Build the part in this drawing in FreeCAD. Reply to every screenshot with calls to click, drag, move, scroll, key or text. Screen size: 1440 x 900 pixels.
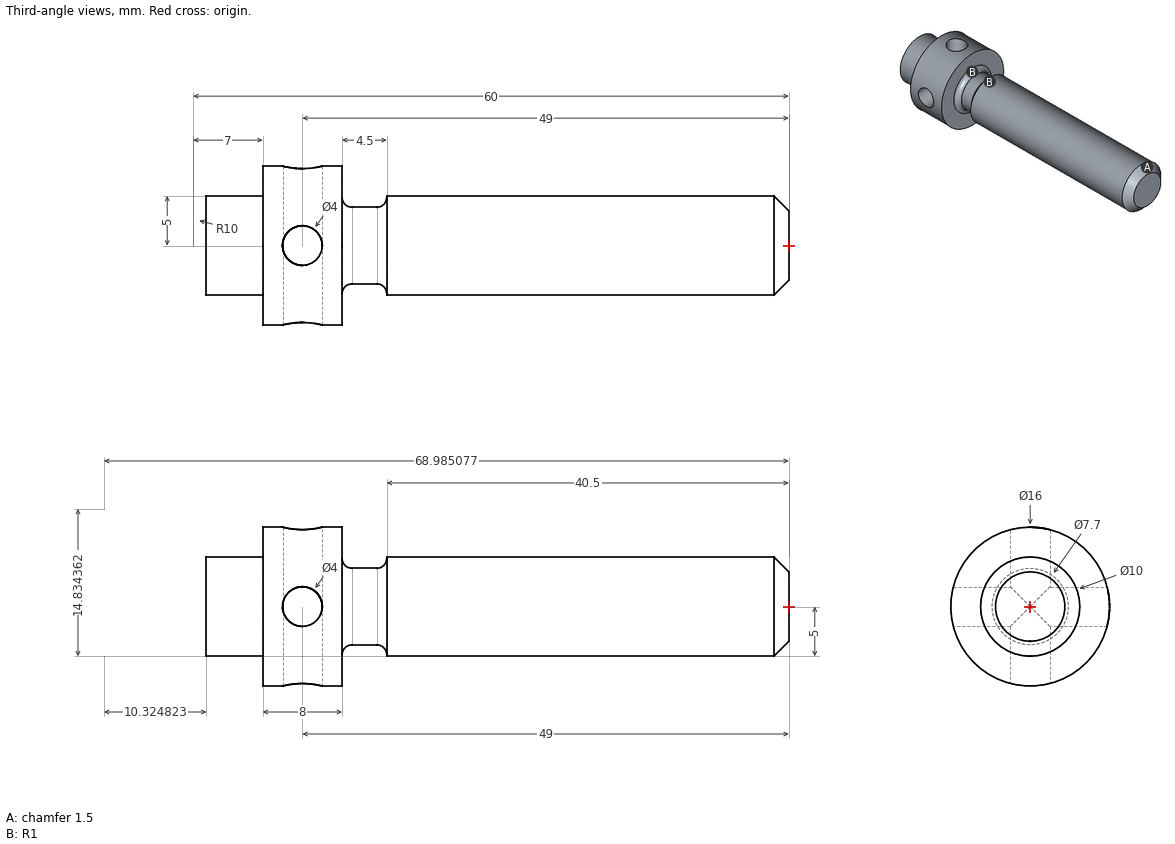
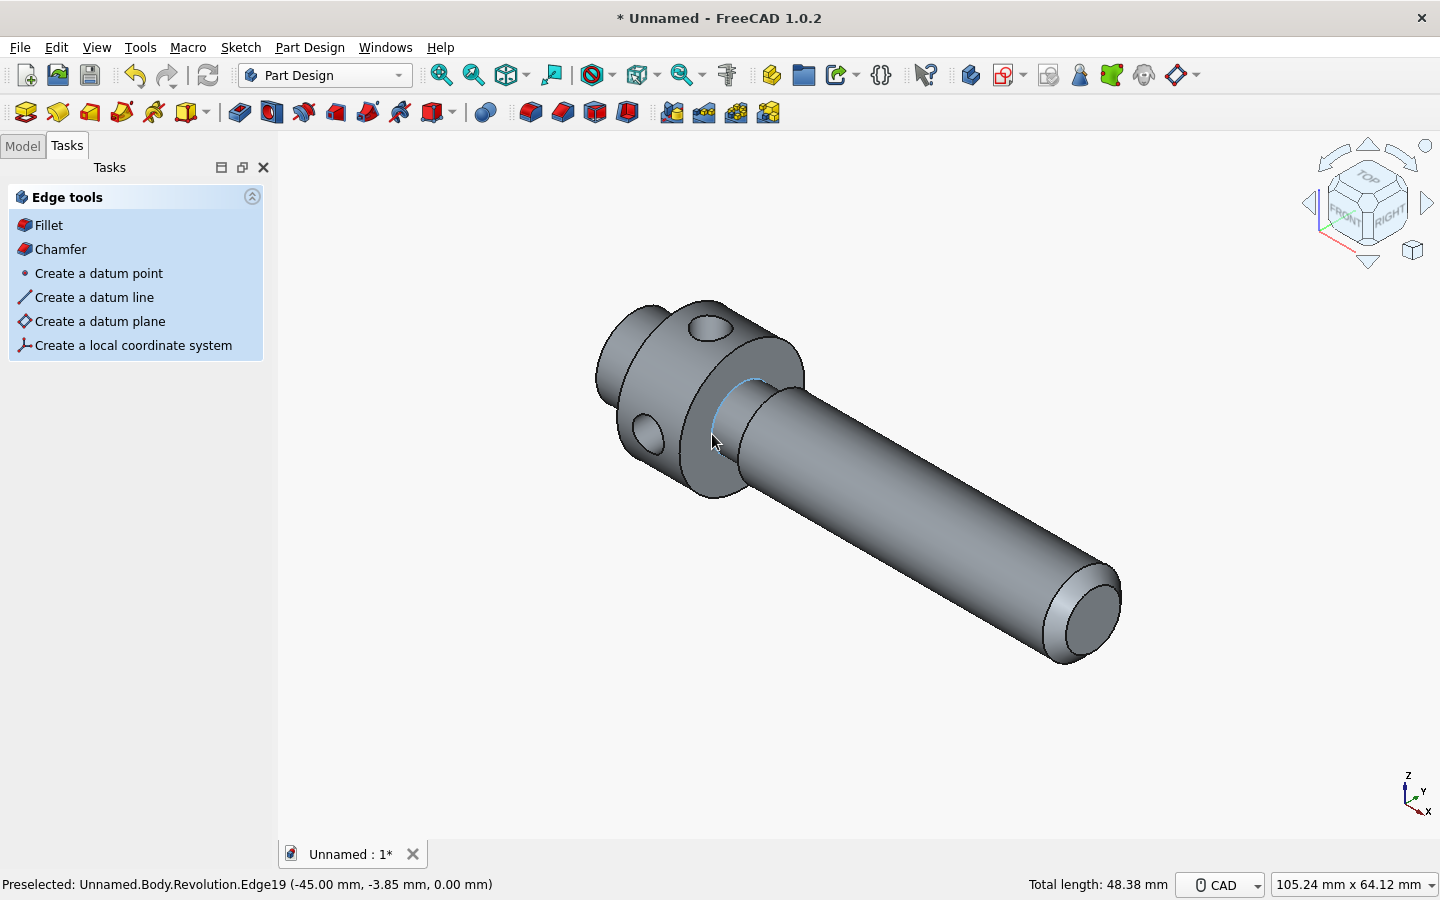
click(532, 112)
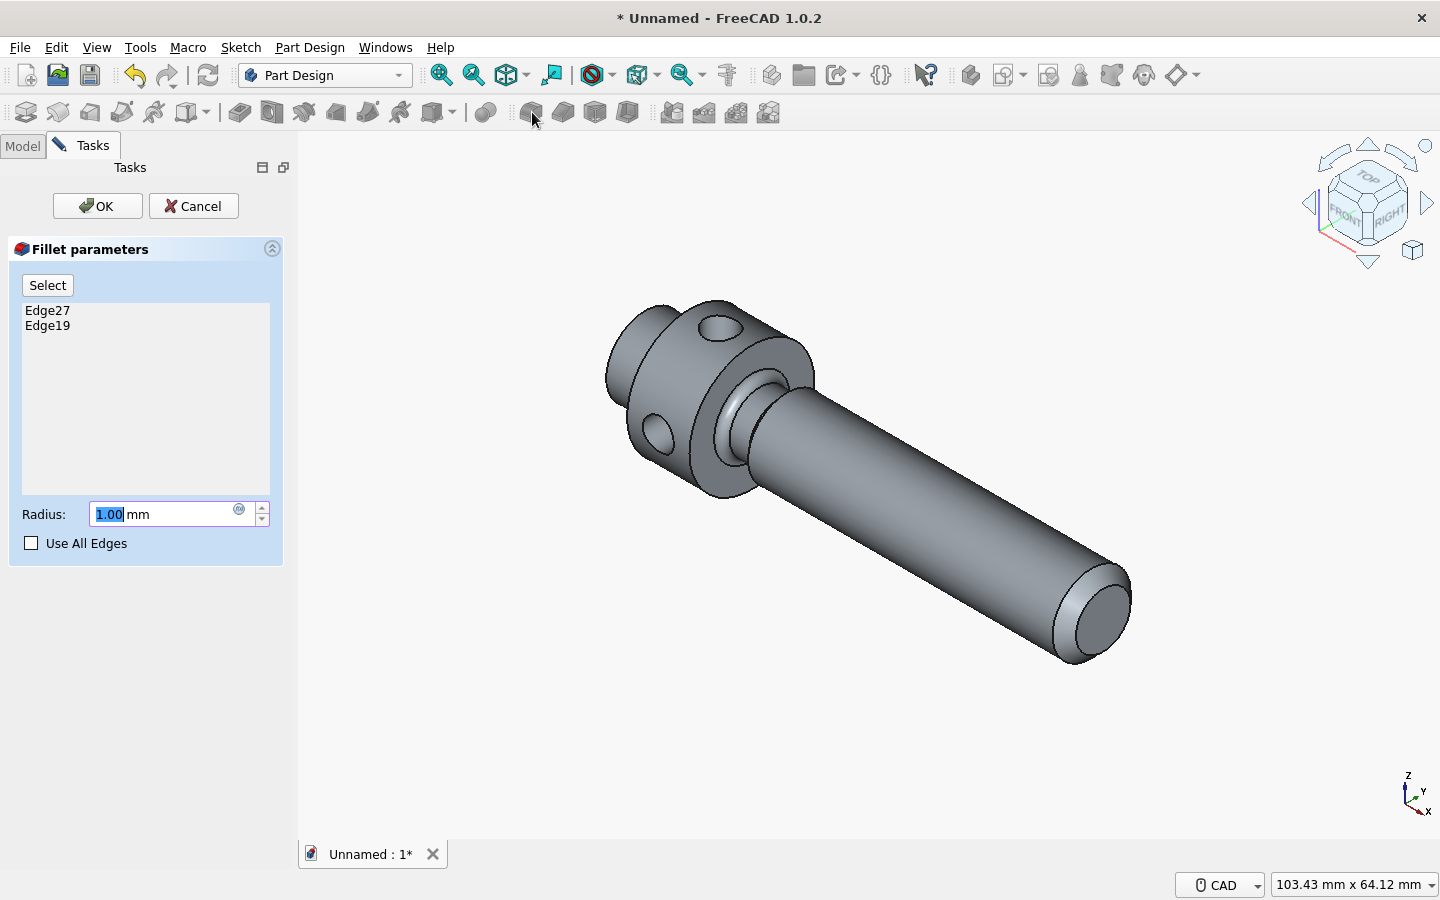
text(1)
key(Tab)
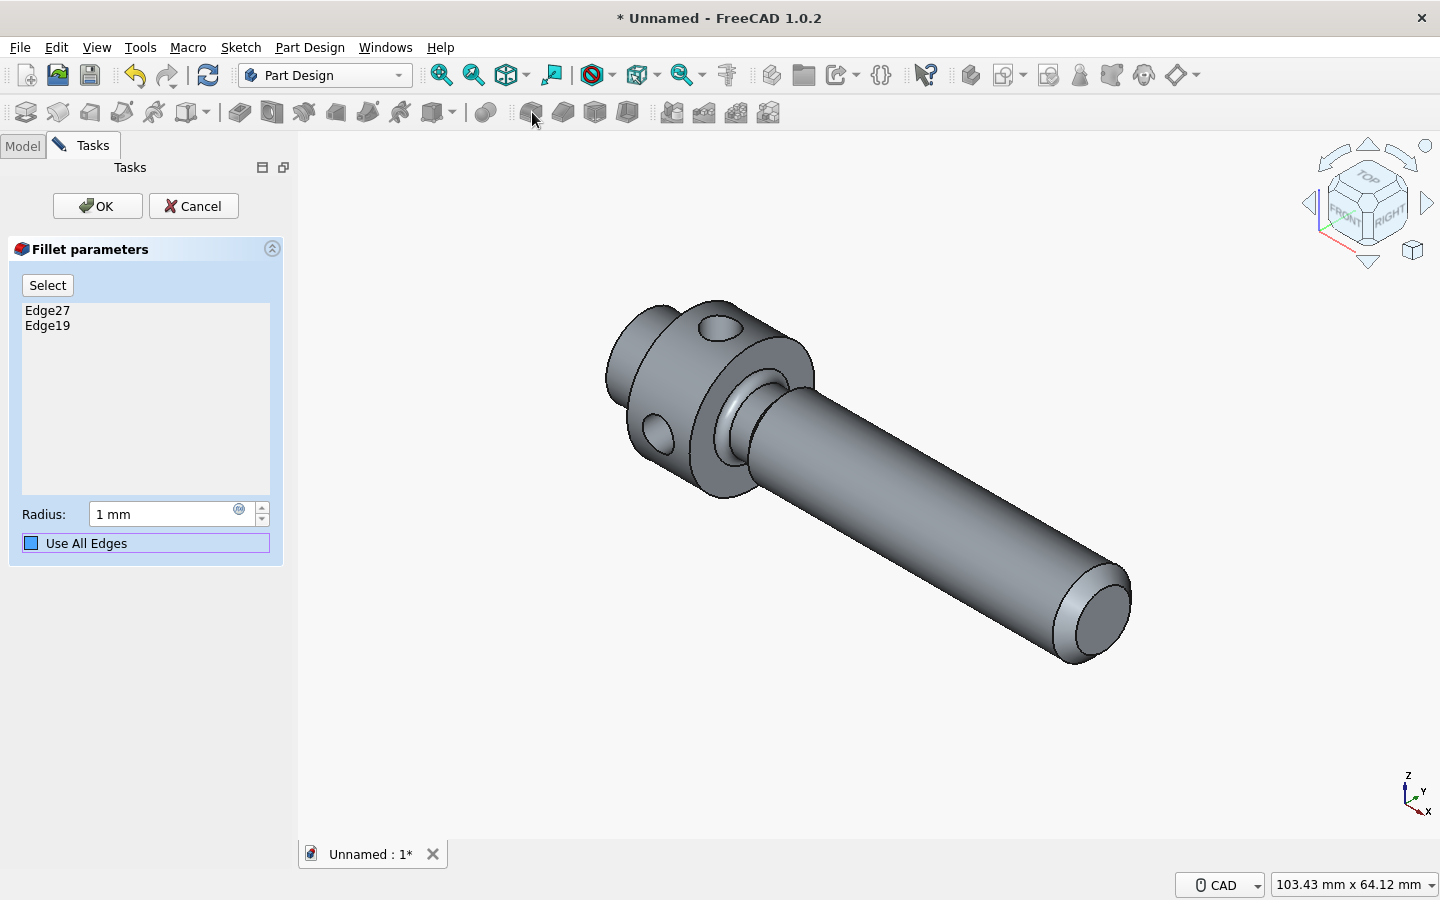
click(98, 206)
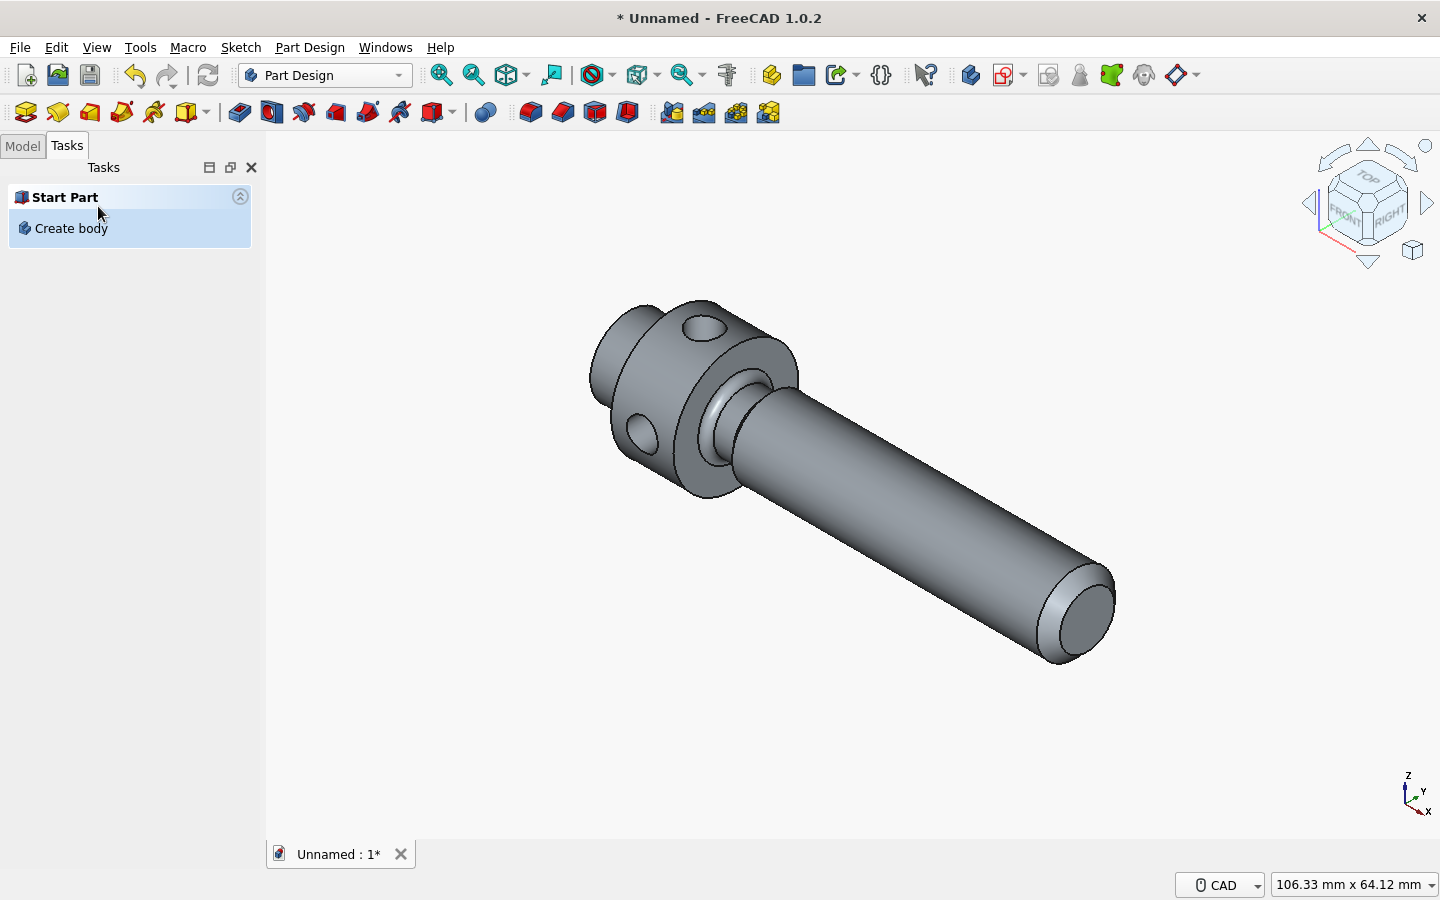
click(1004, 76)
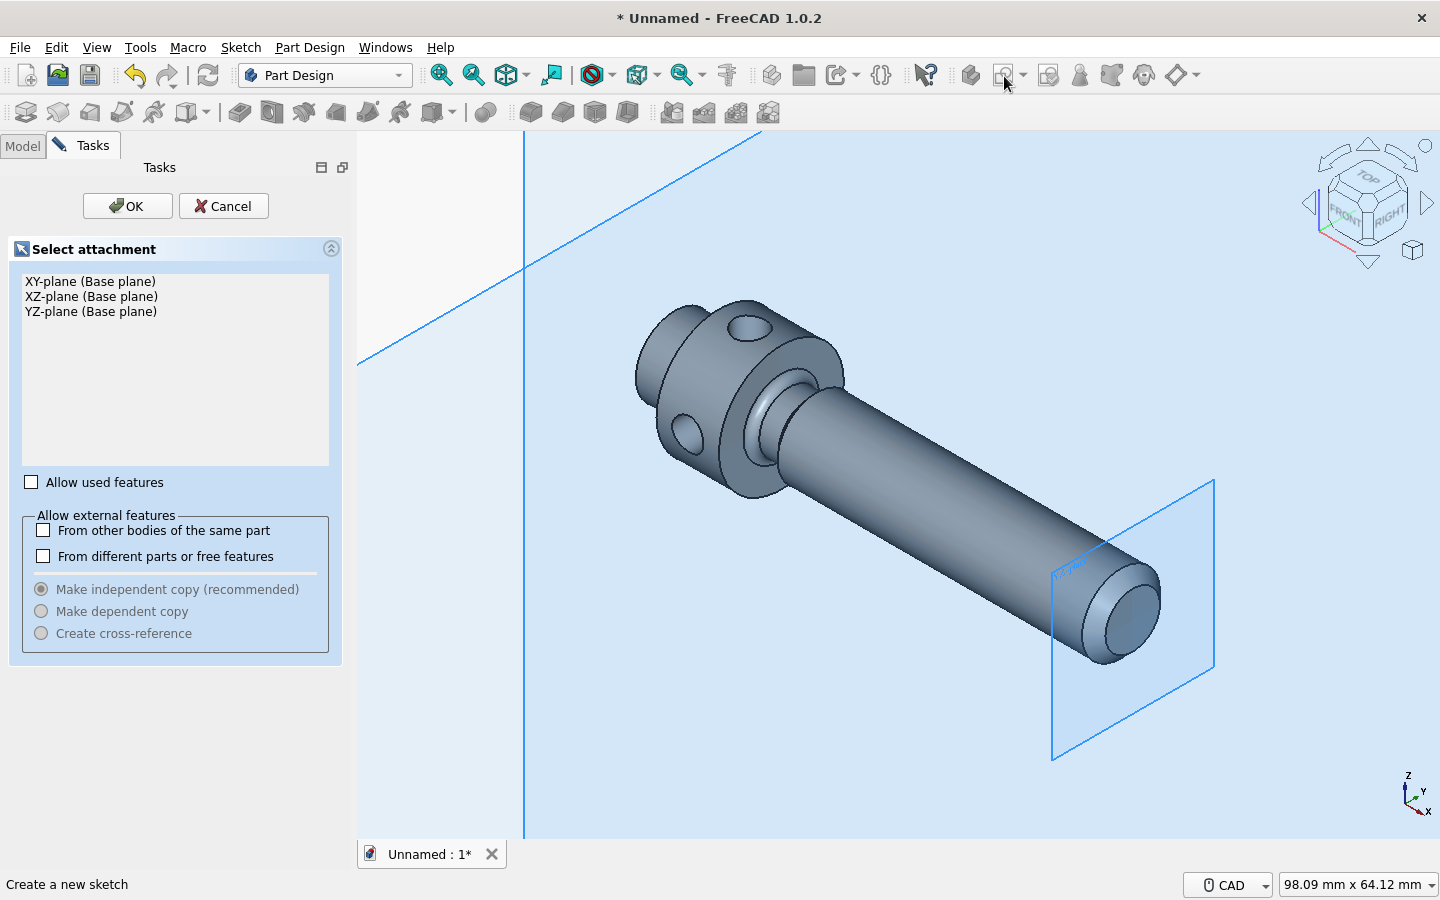
click(82, 296)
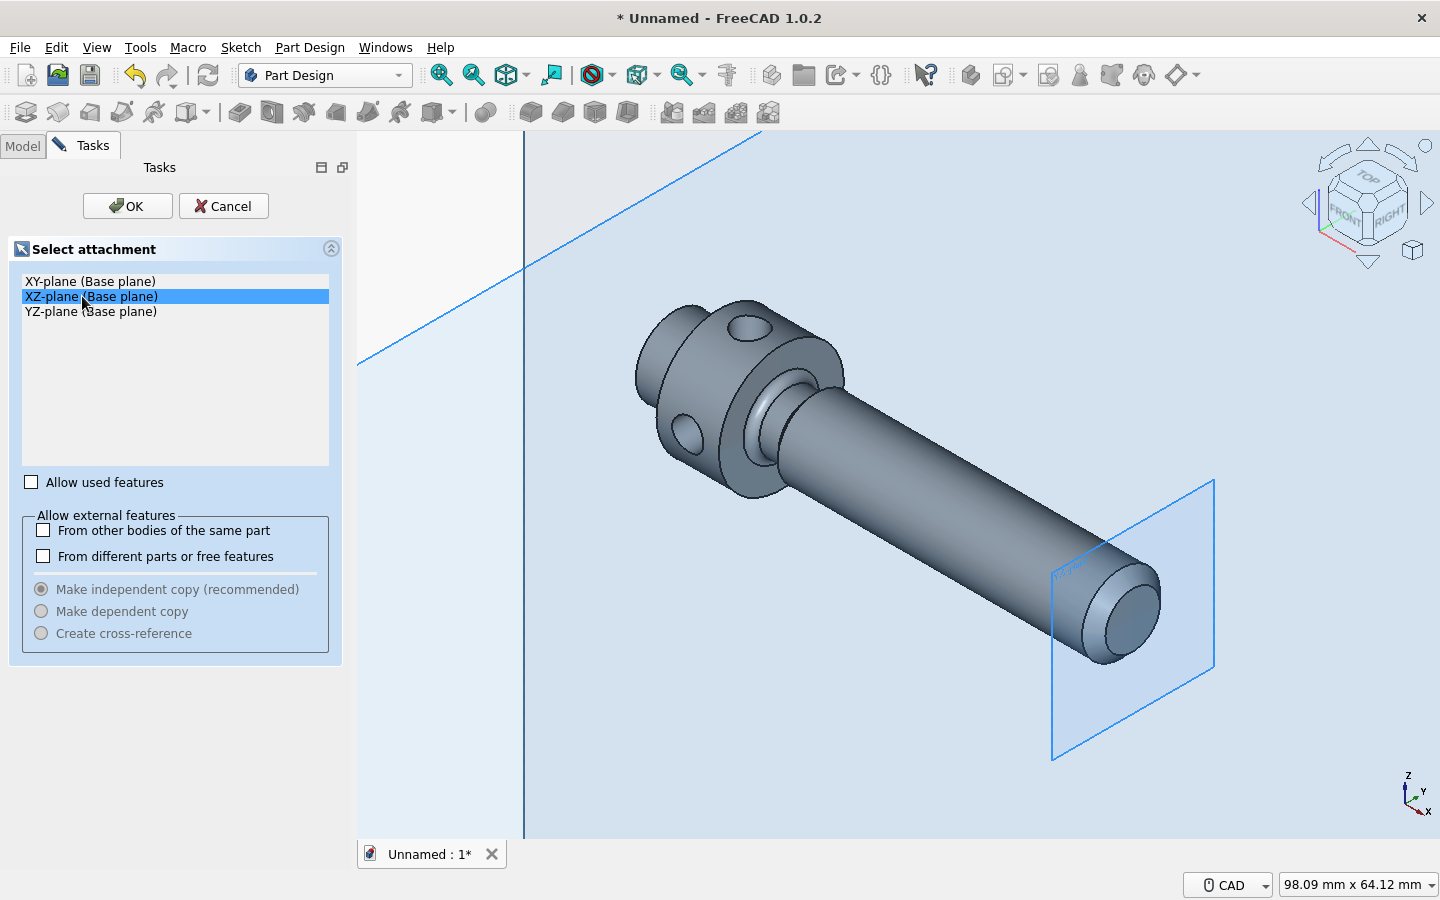
click(128, 206)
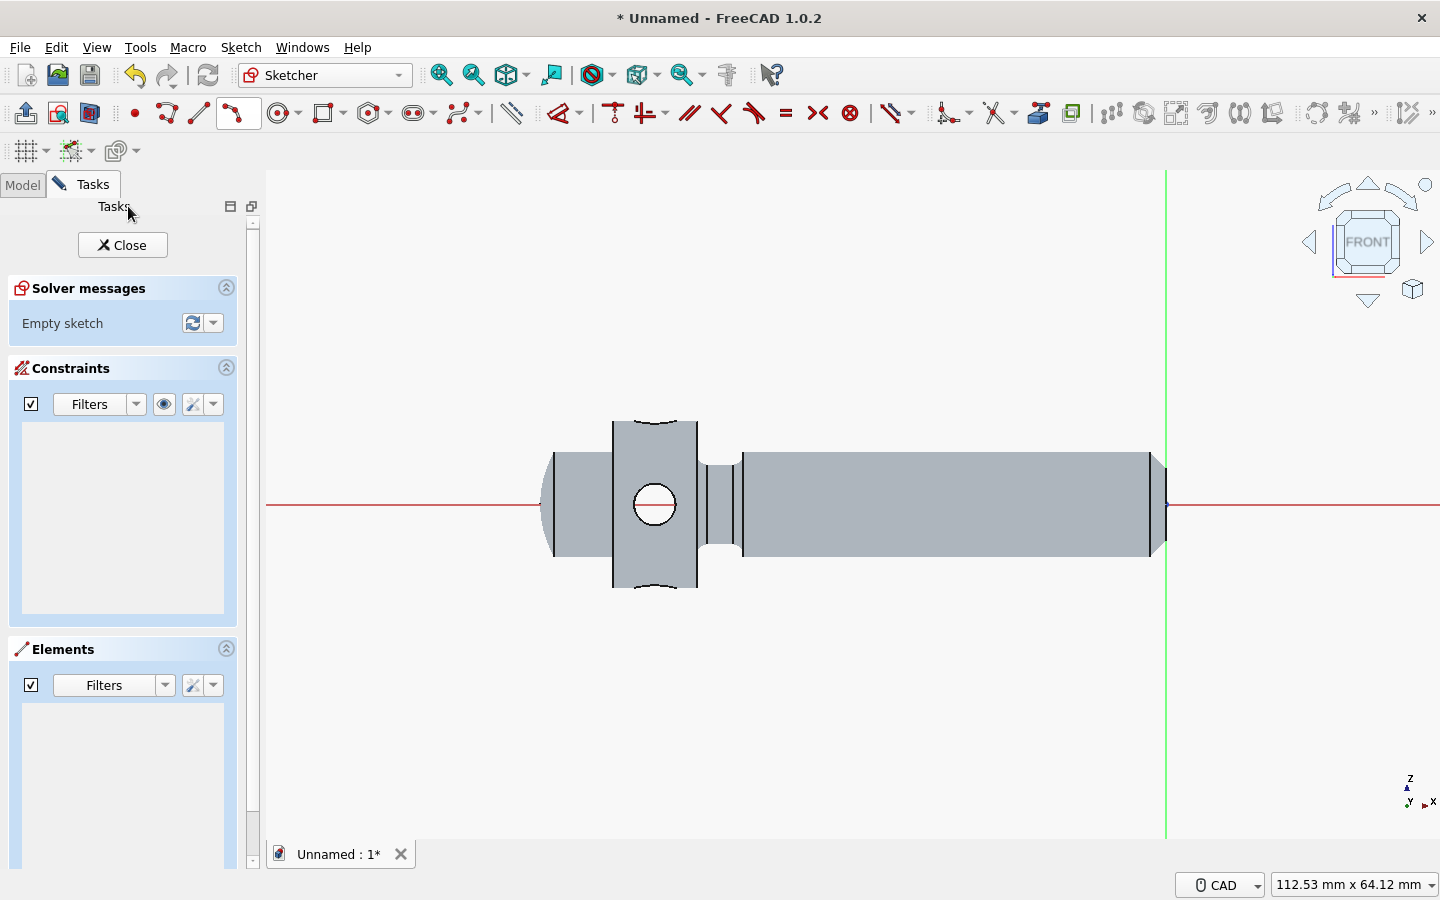
click(90, 114)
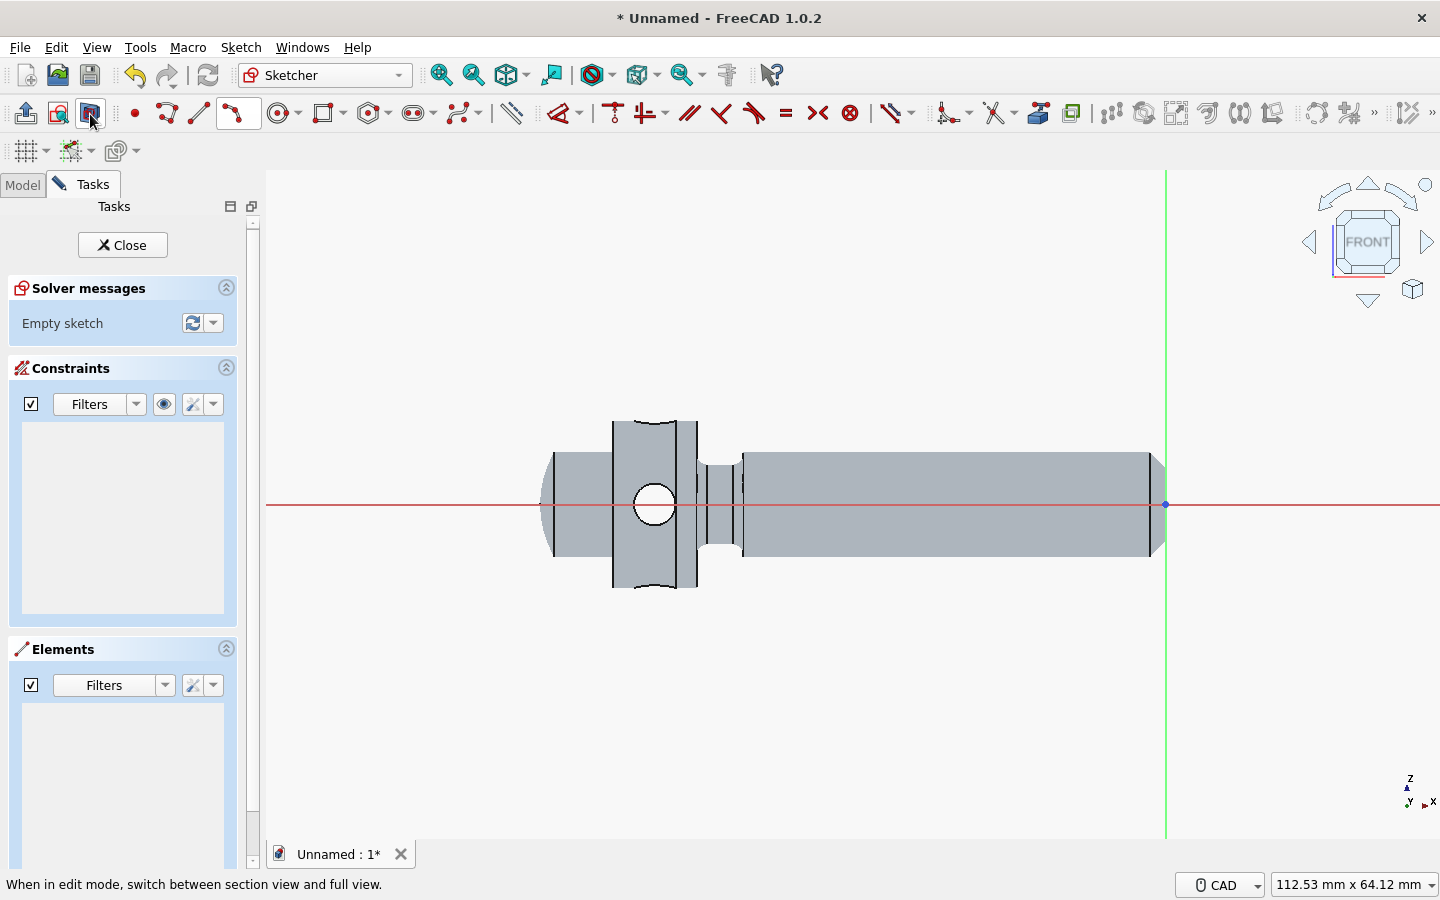
scroll(335, 465, up, 5)